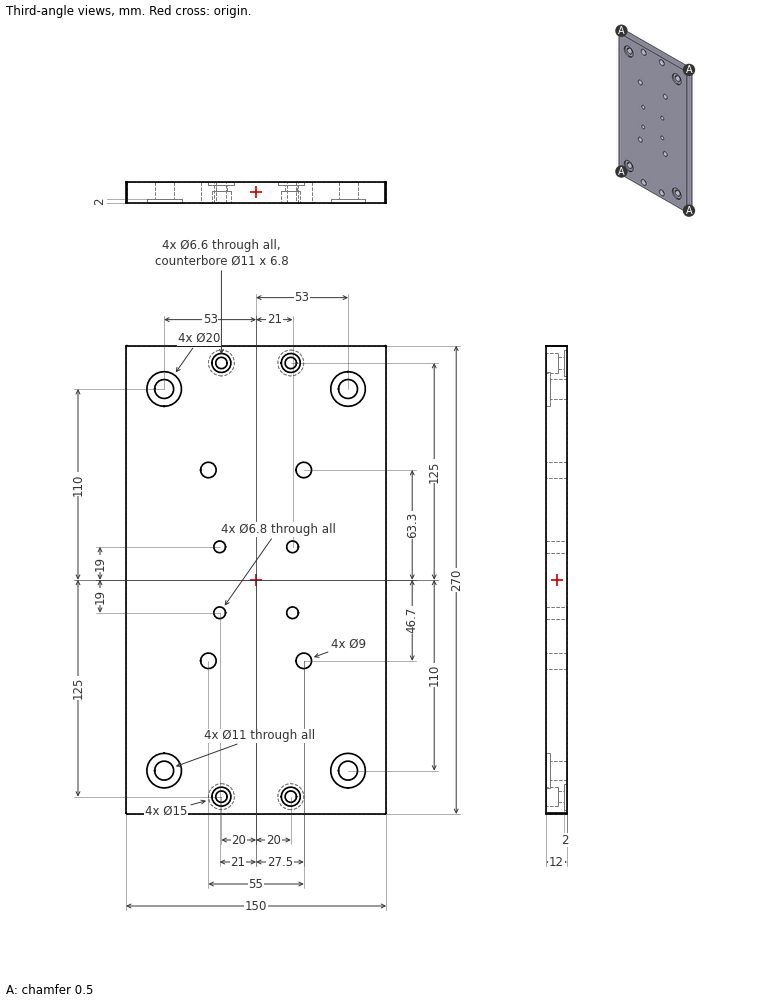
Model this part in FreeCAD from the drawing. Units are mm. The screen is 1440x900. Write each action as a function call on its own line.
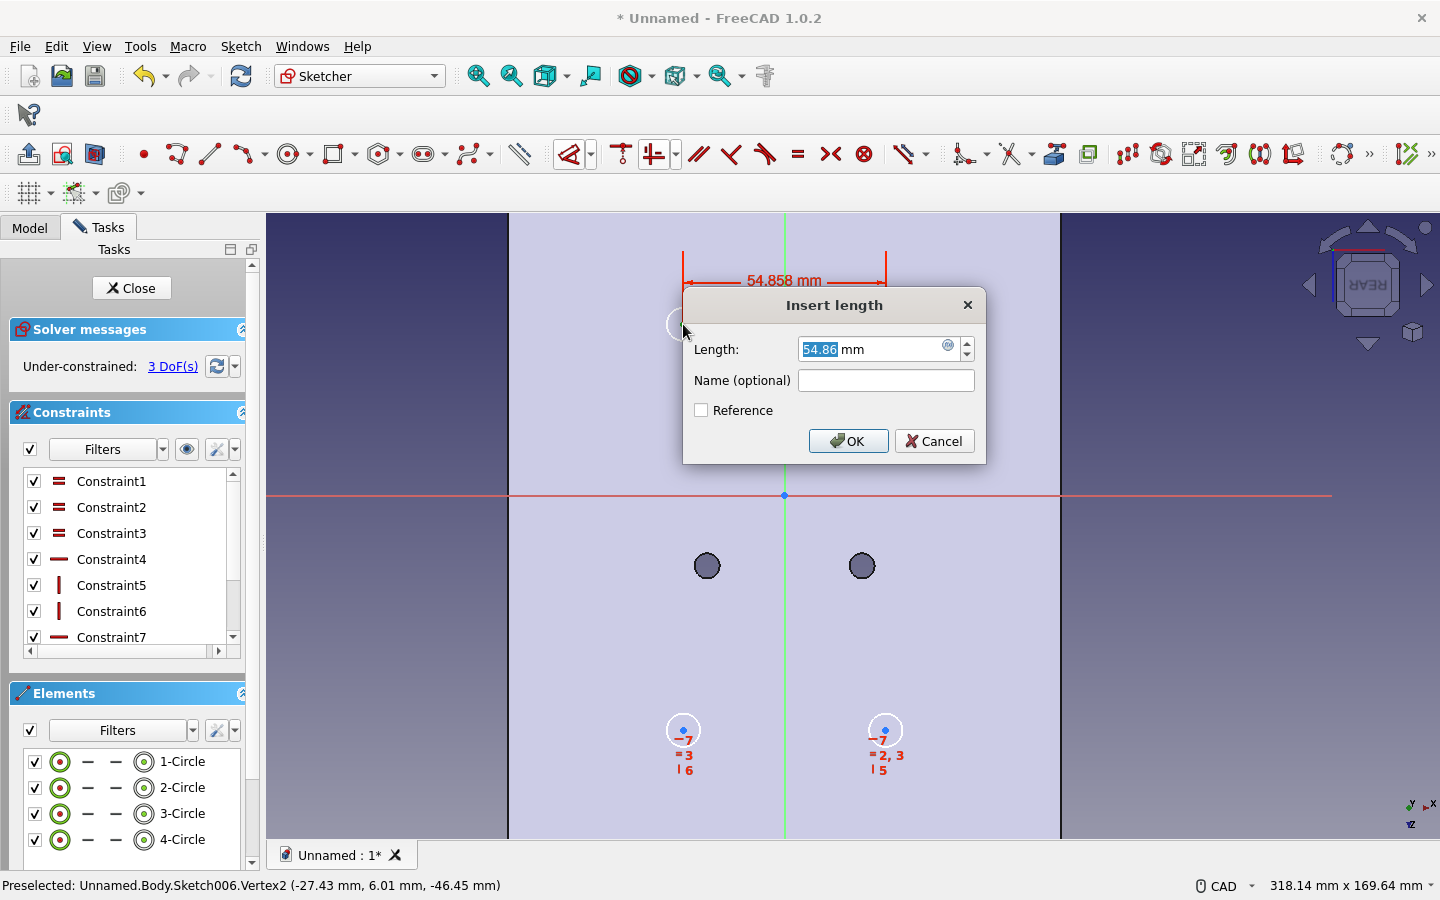
text(55)
key(Return)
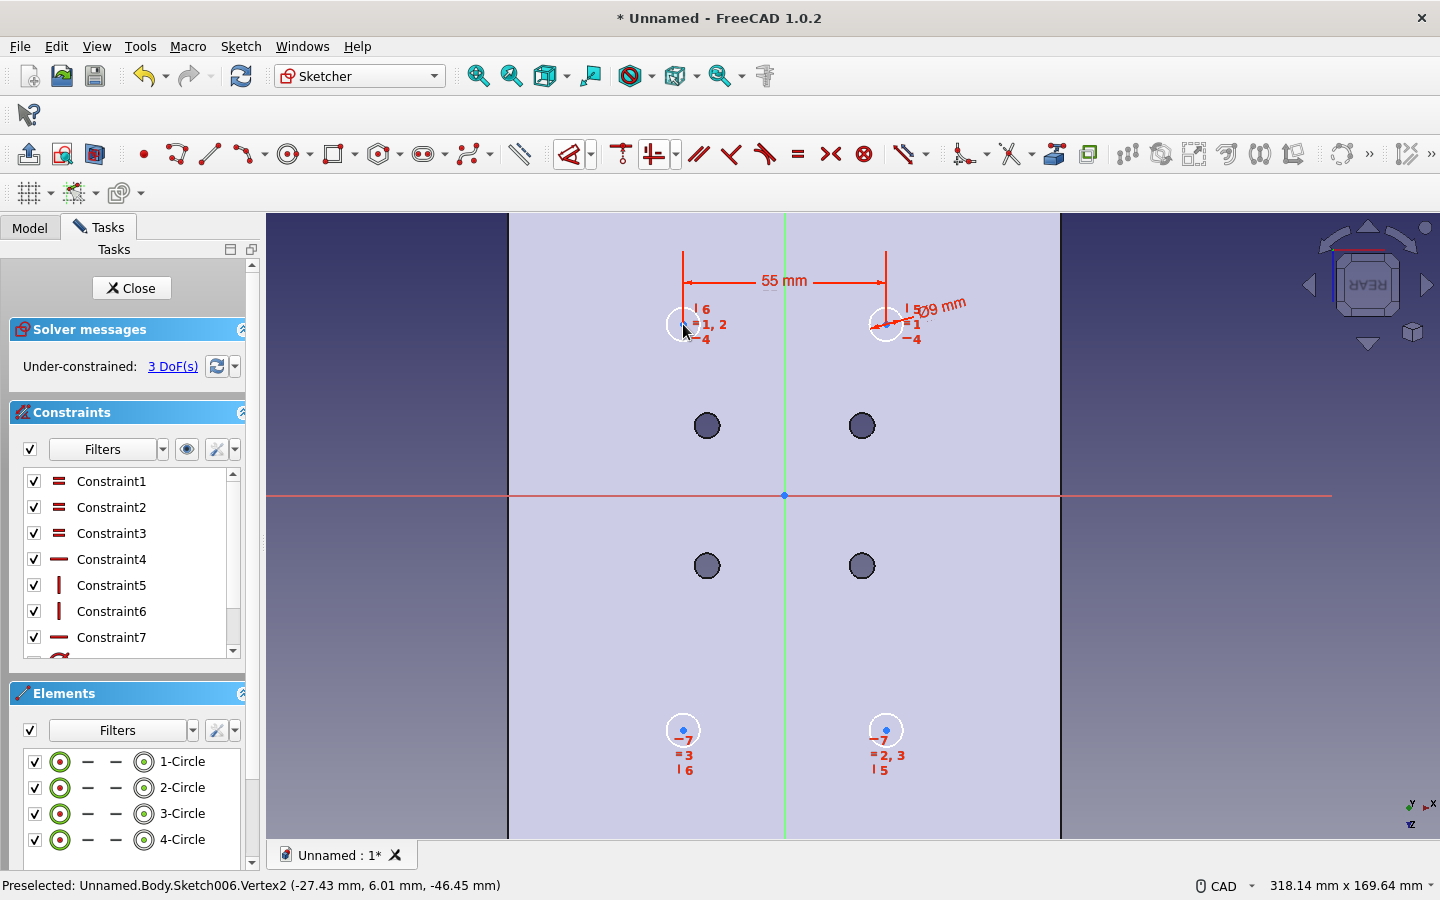
click(886, 324)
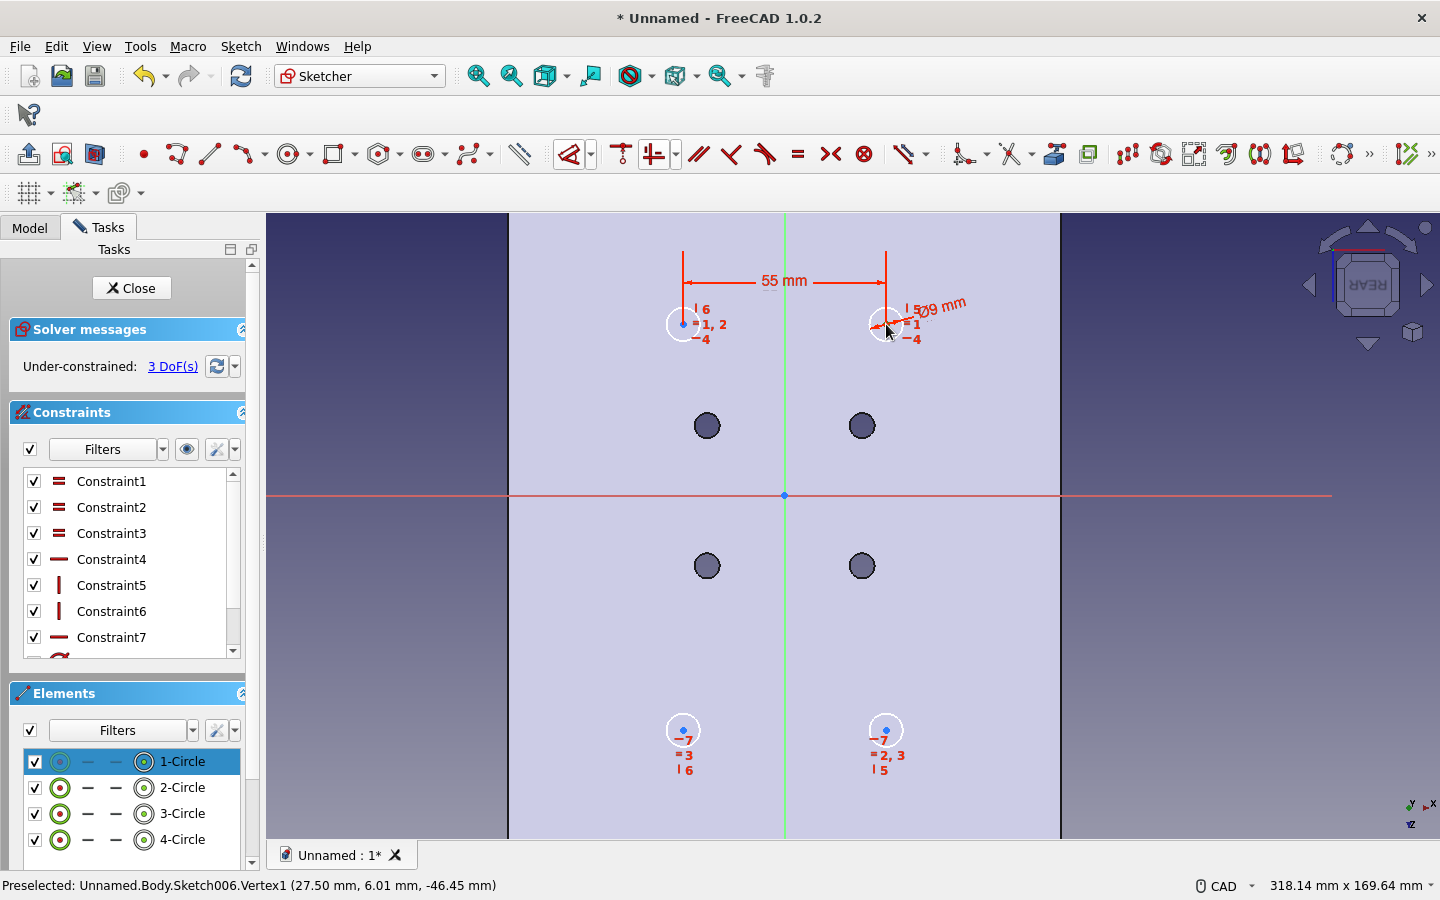
key(l)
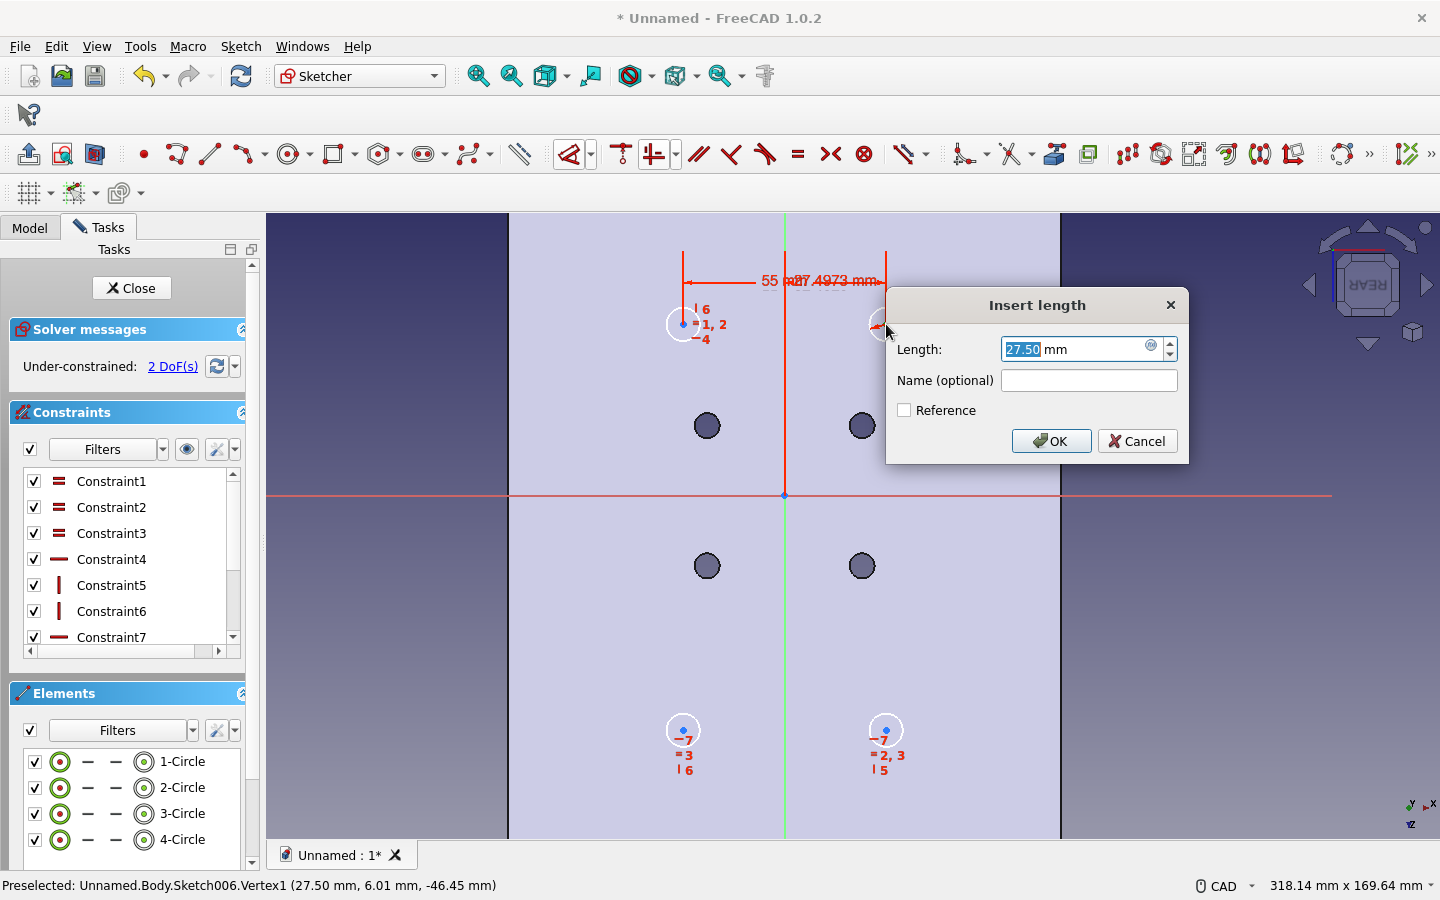
text(27.5)
key(Return)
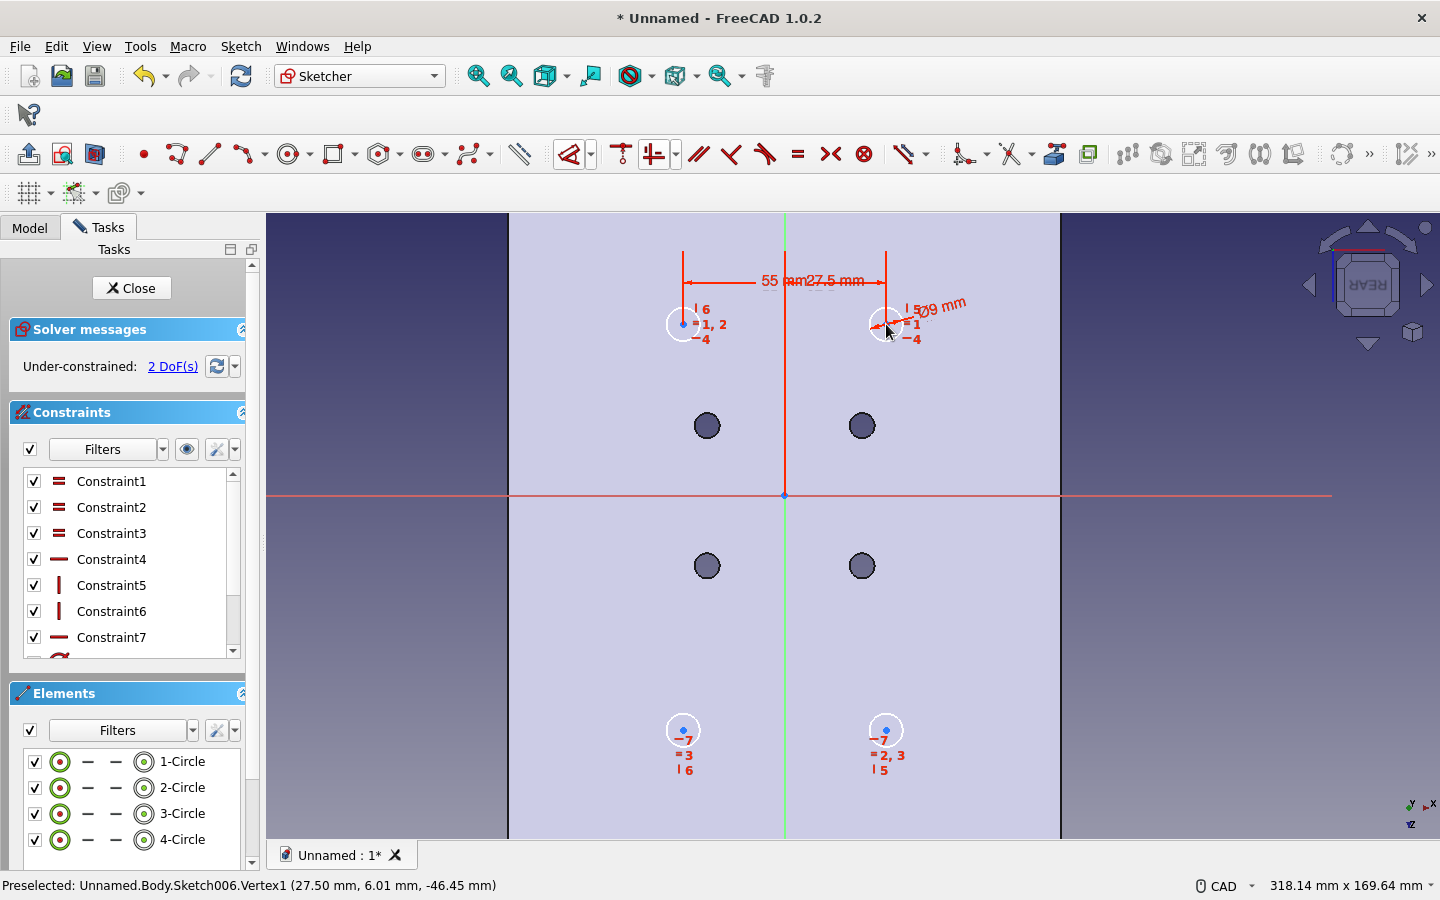
click(886, 324)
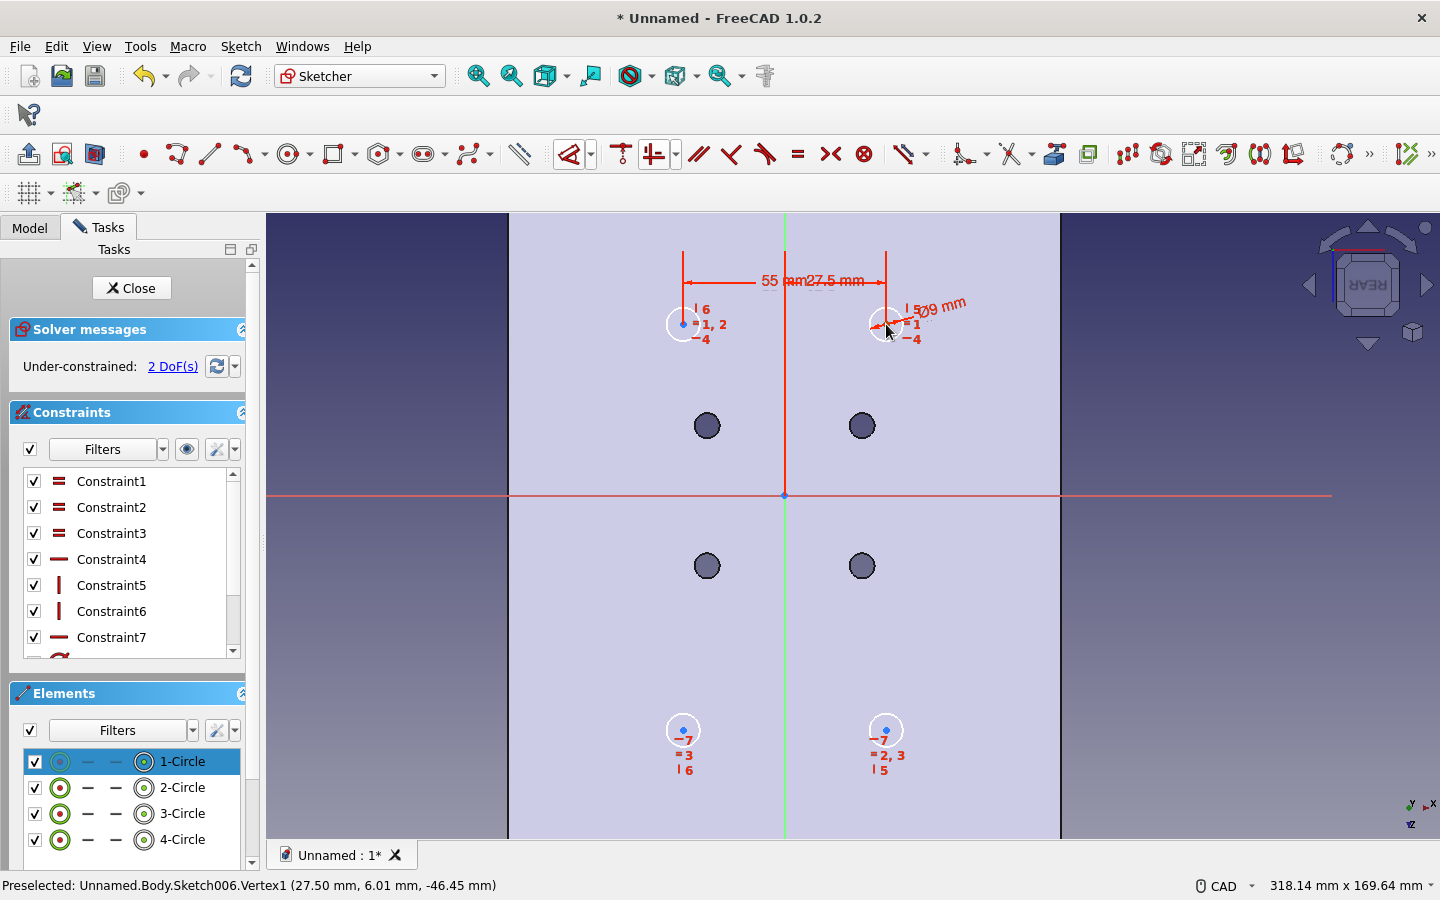
key(i)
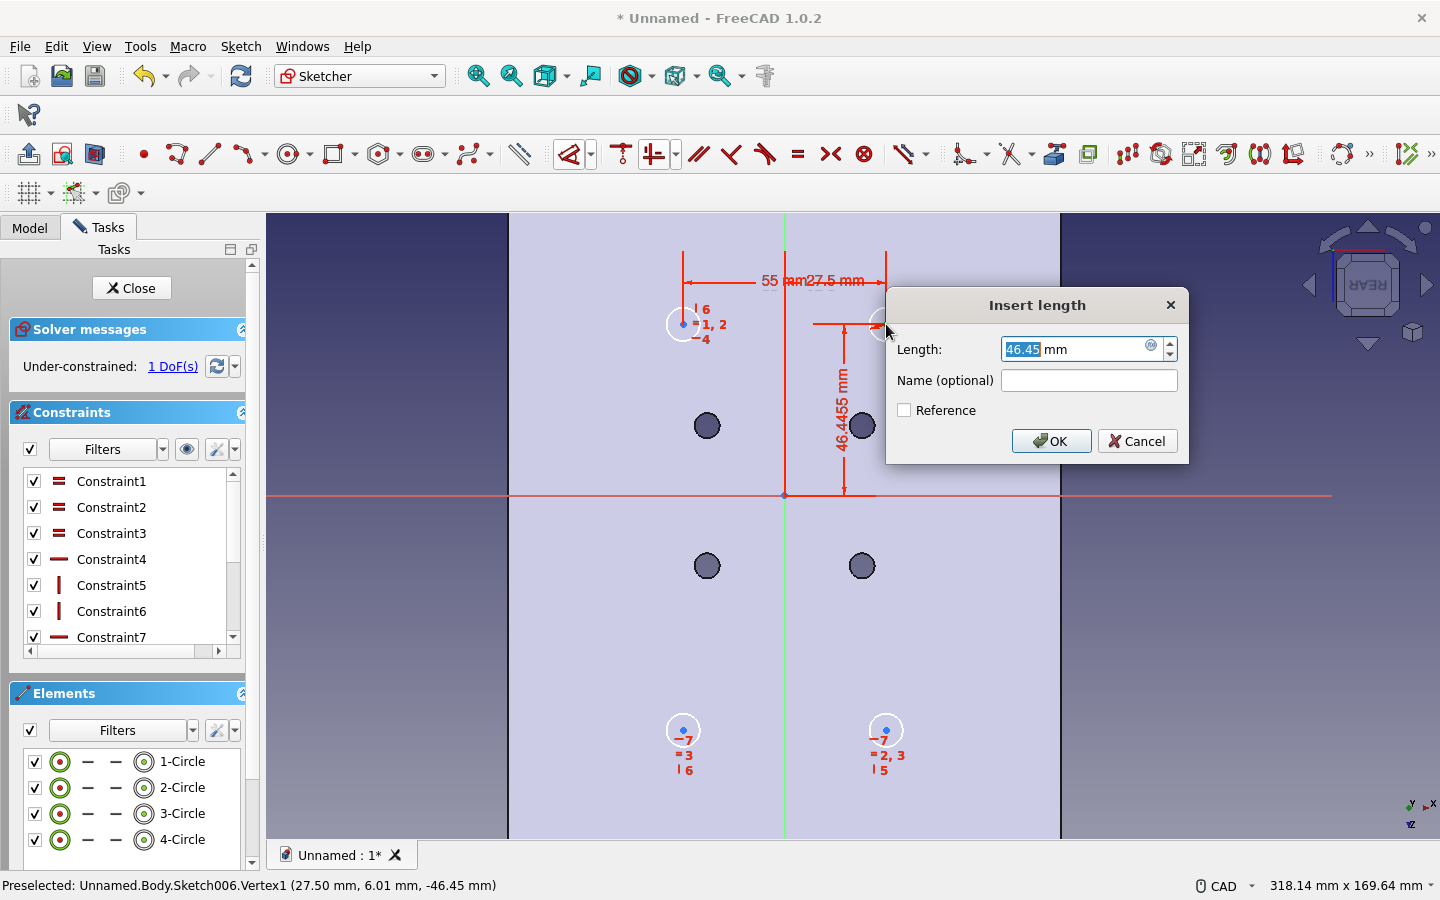
text(46.7)
key(Return)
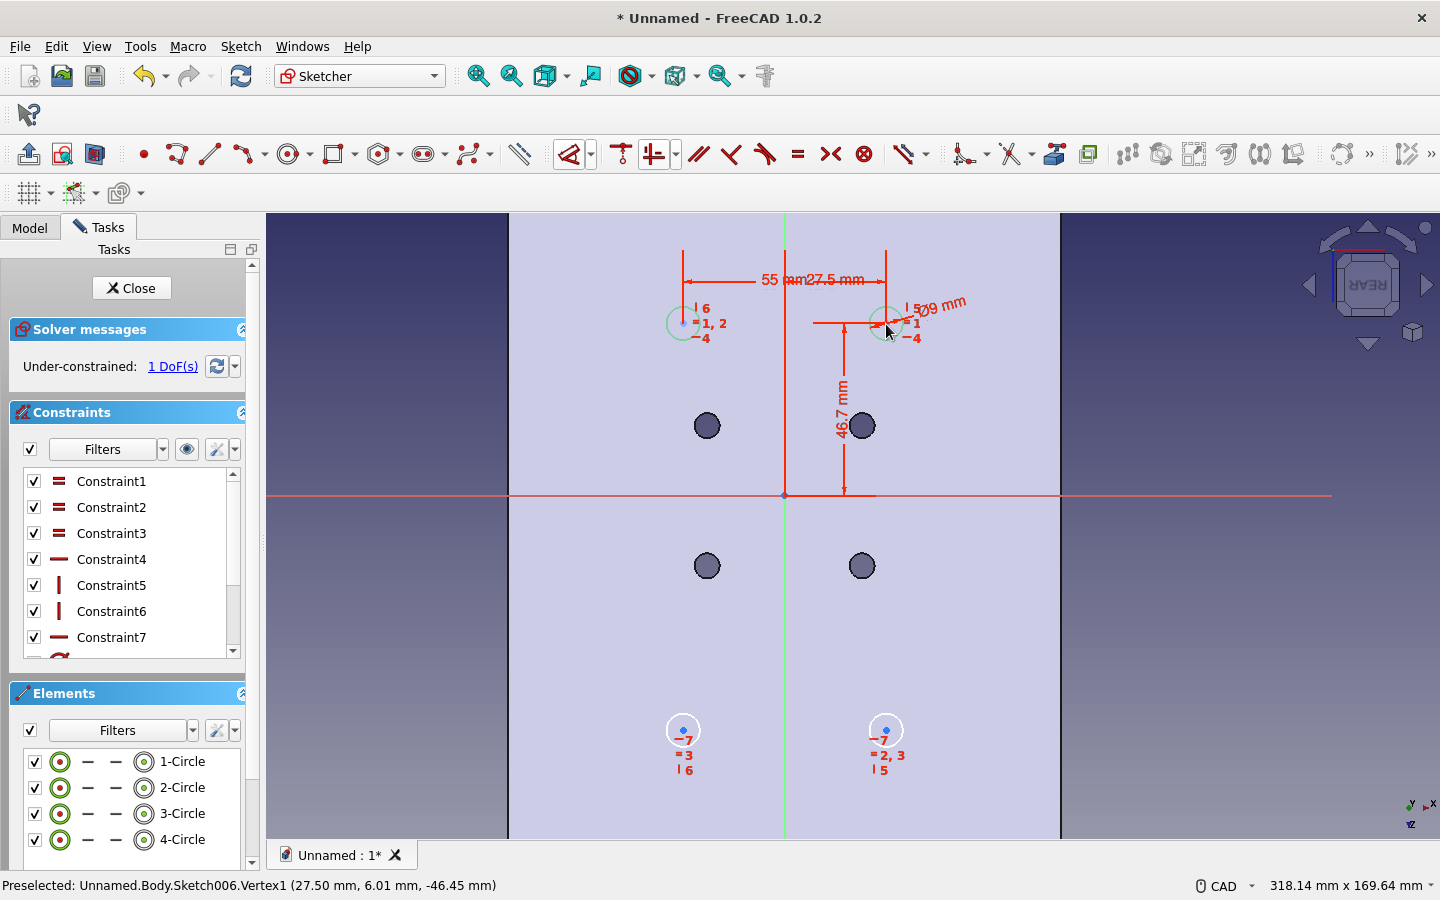
click(886, 730)